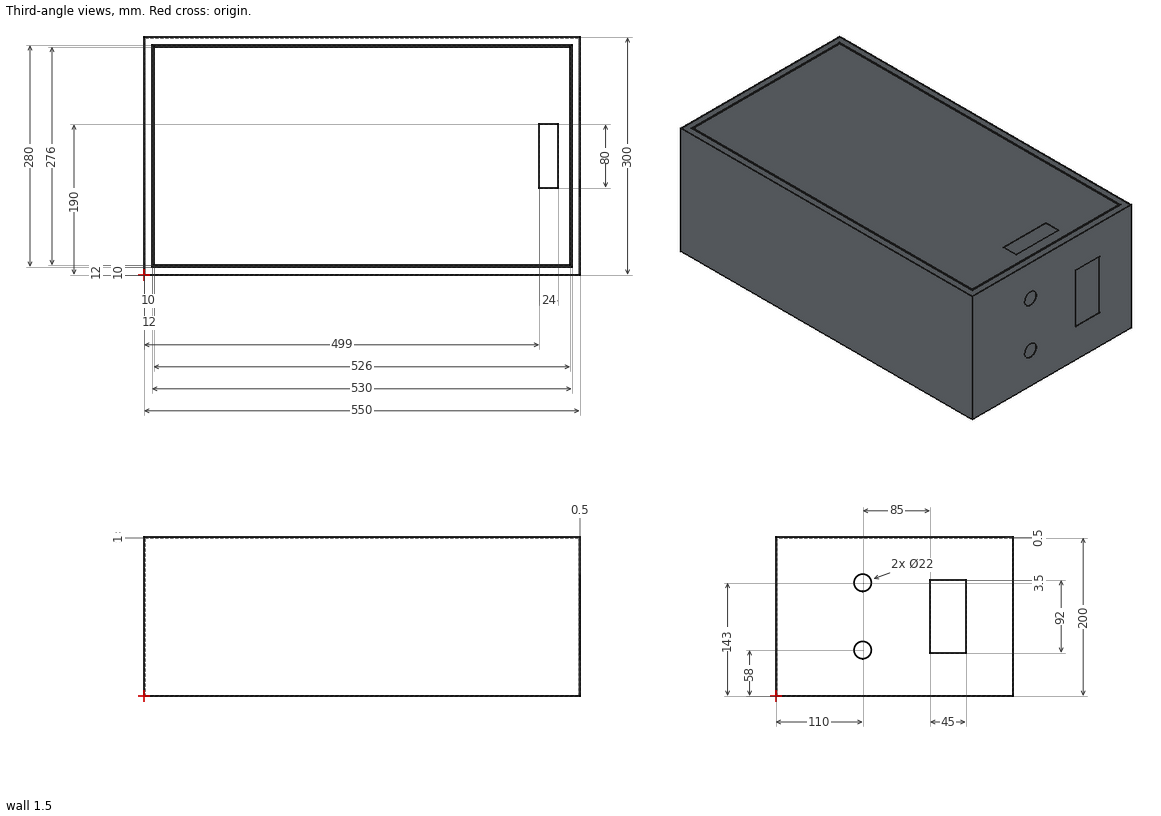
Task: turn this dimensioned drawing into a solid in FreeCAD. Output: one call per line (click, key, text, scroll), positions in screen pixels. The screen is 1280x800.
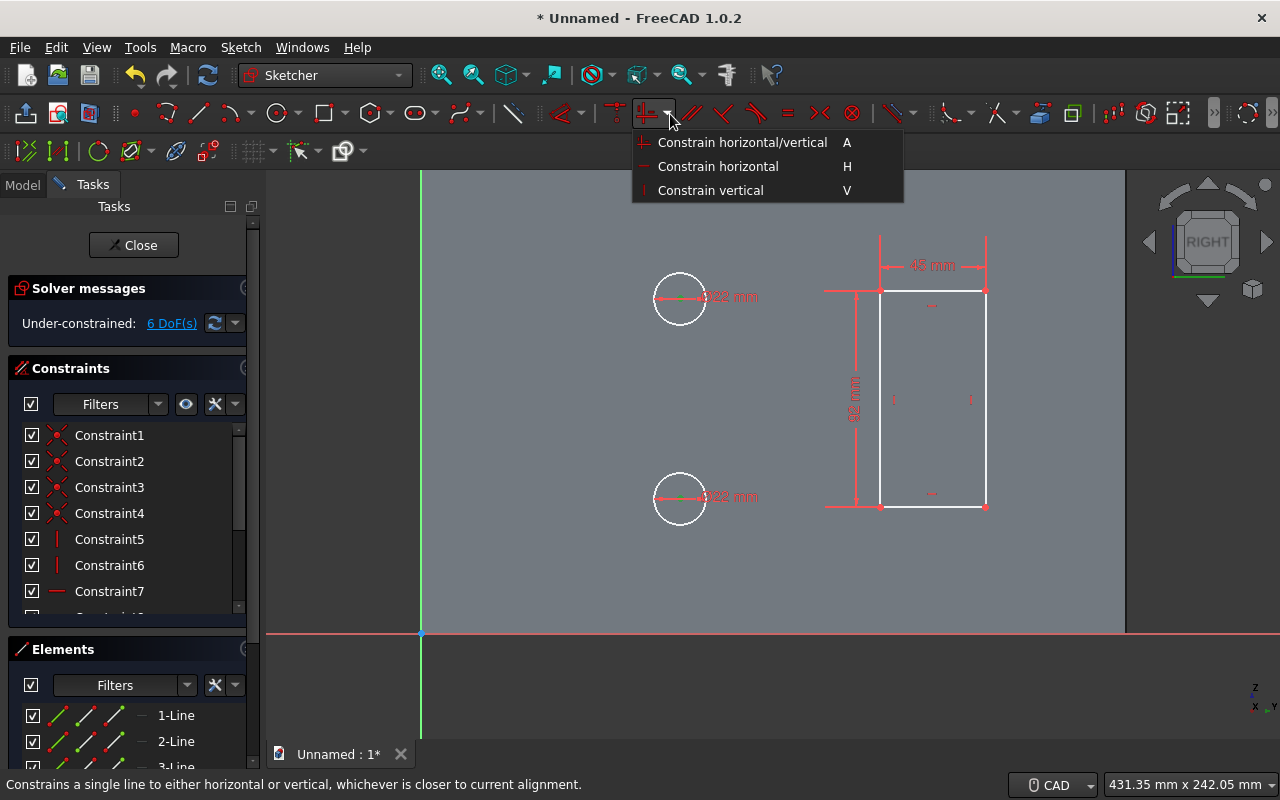
click(768, 190)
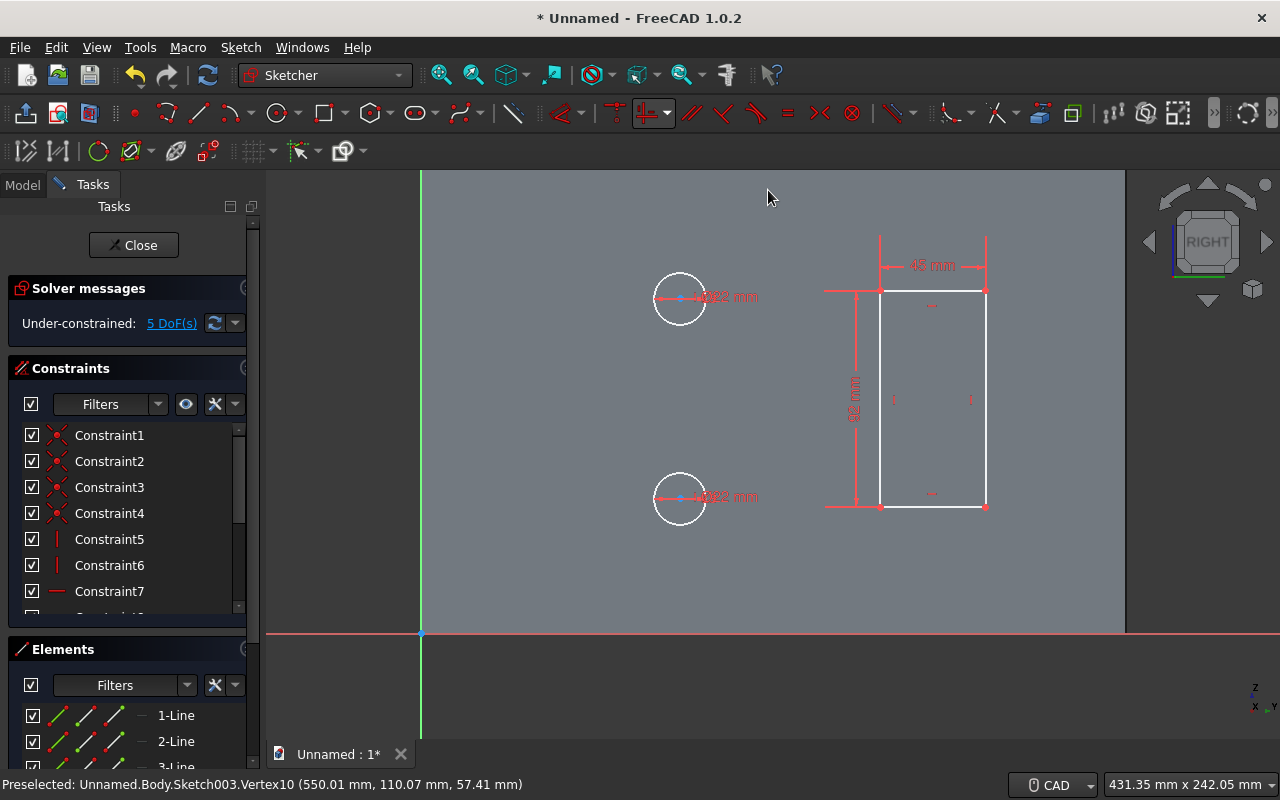
click(560, 114)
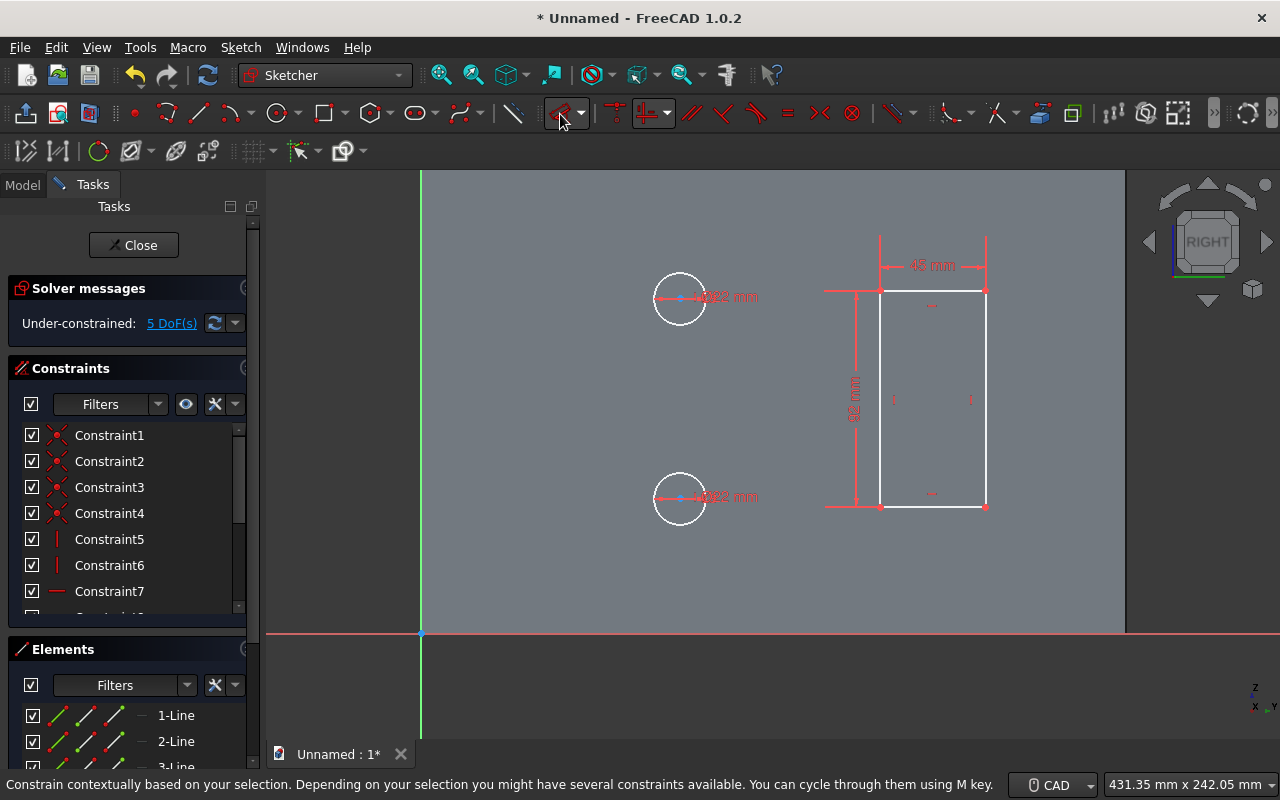
click(680, 499)
click(387, 566)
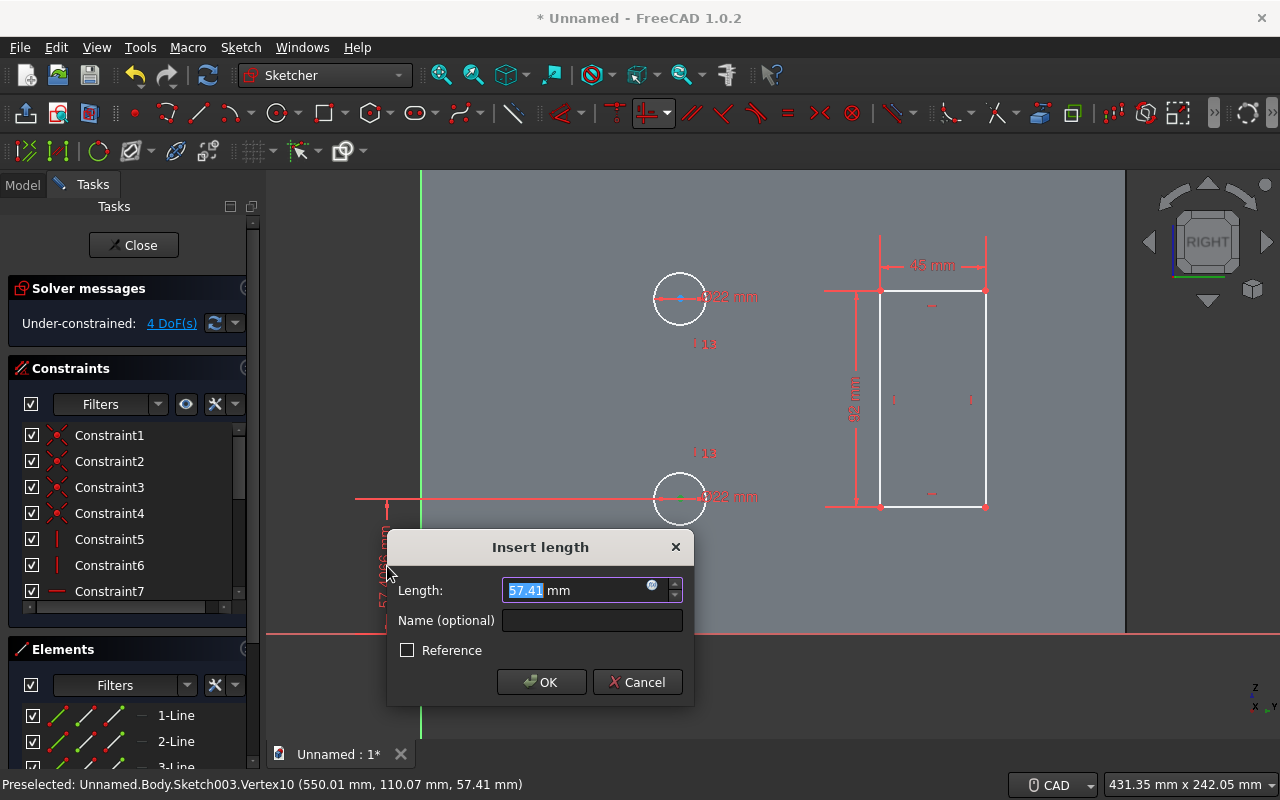
text(58)
key(Return)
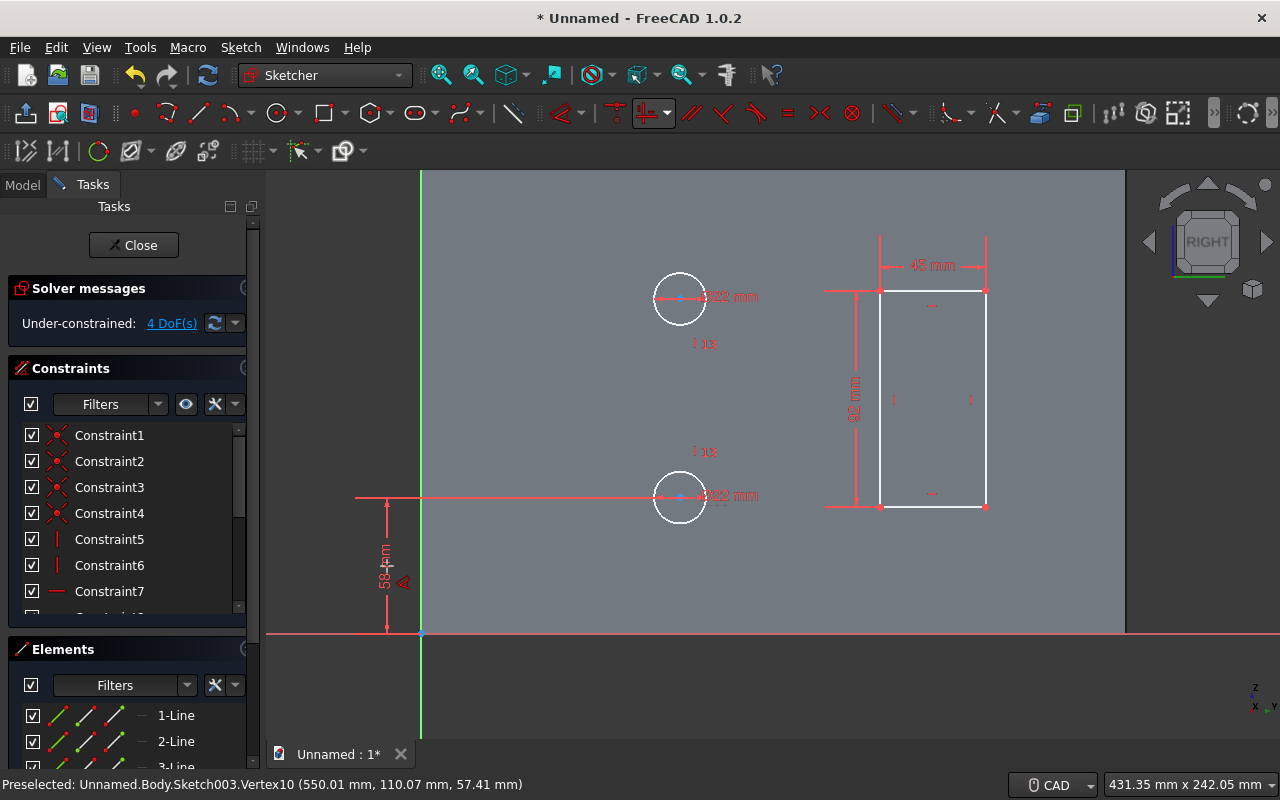
click(680, 299)
click(551, 668)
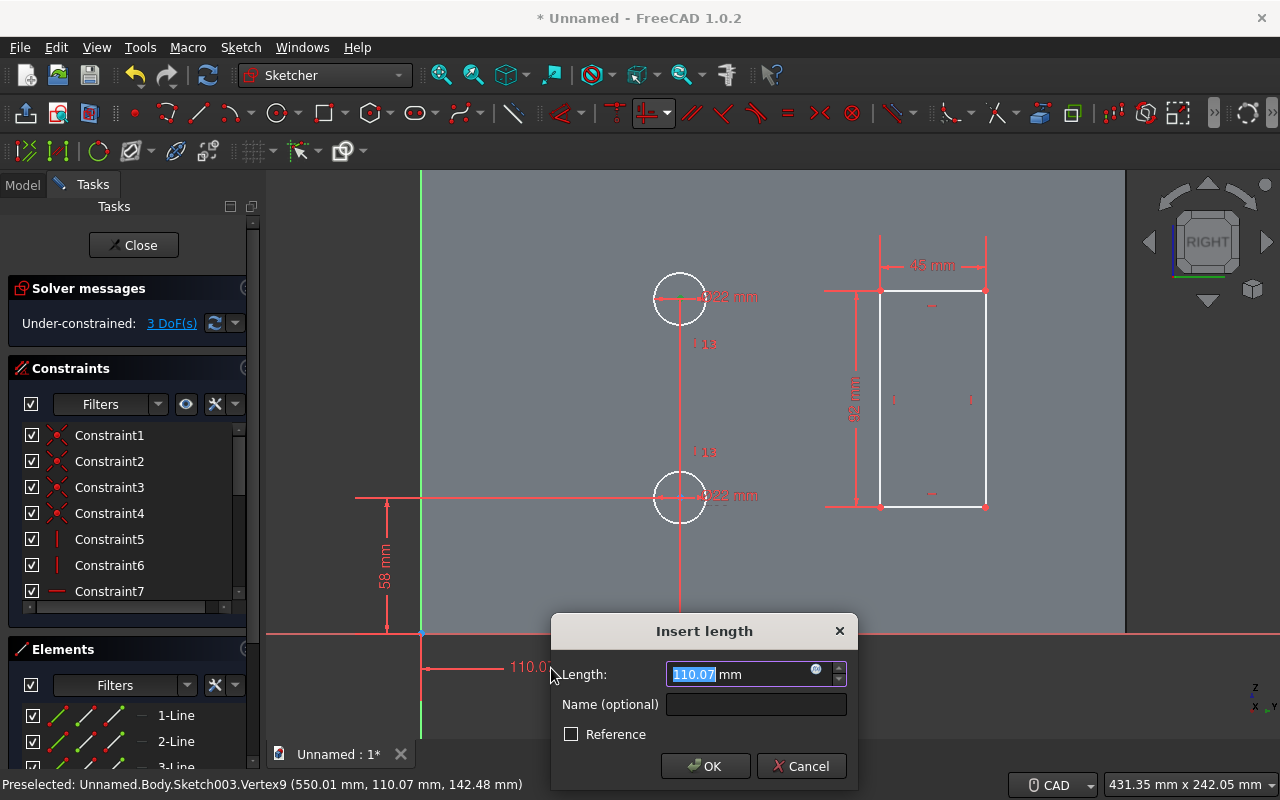
text(110)
key(Return)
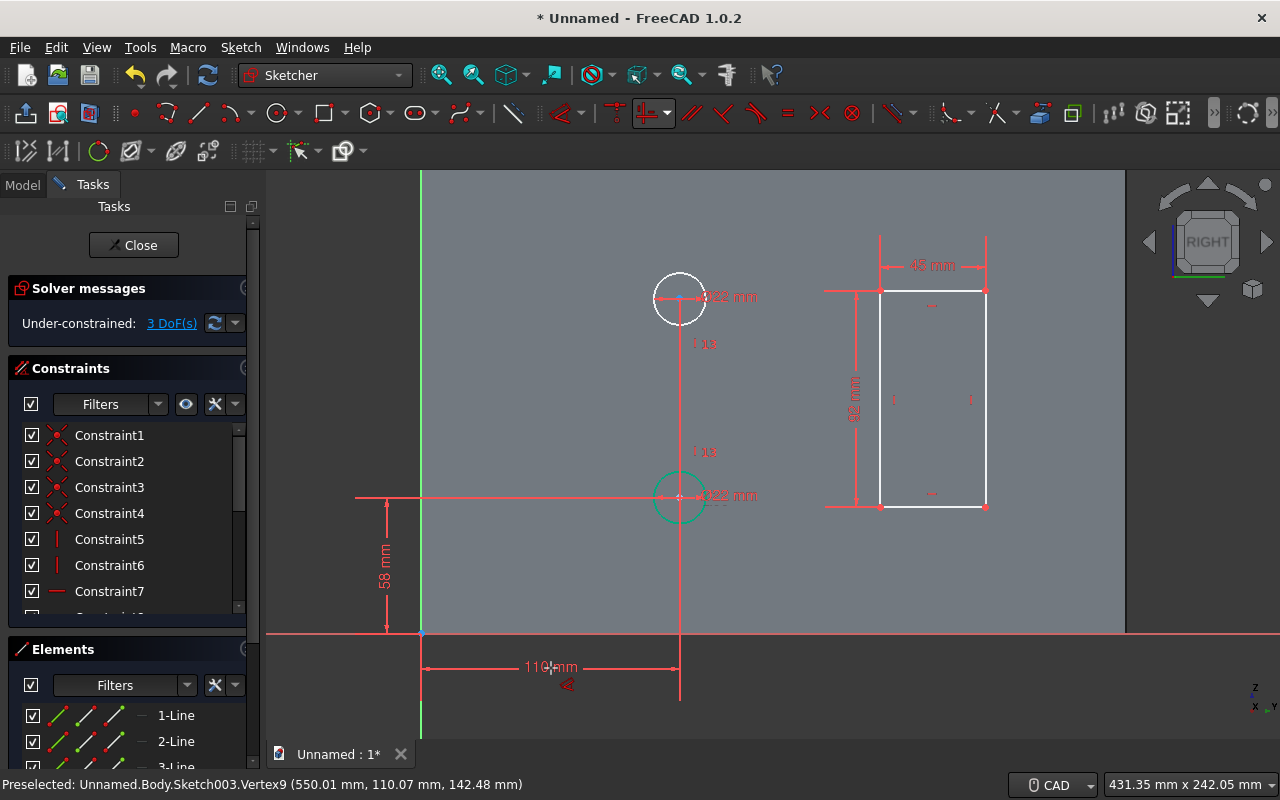
click(680, 299)
click(387, 466)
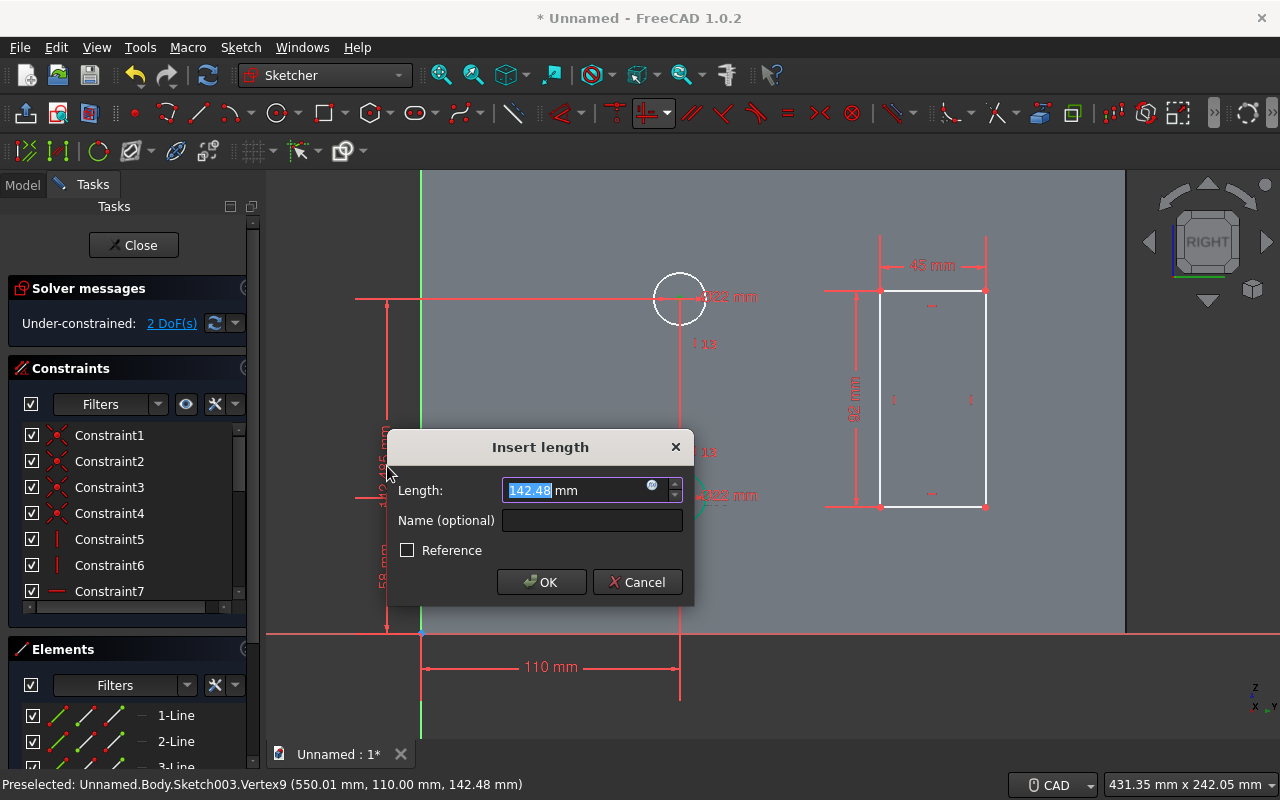
text(143)
key(Return)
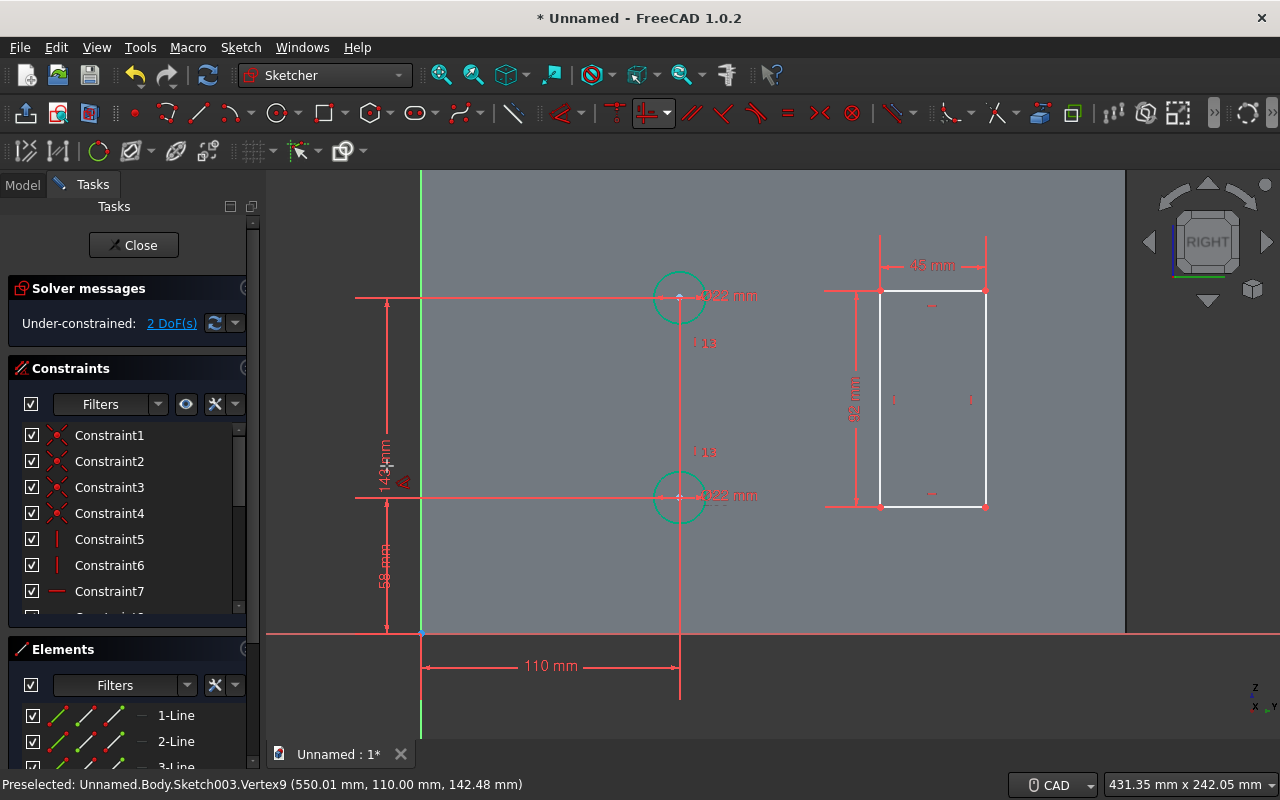
click(880, 291)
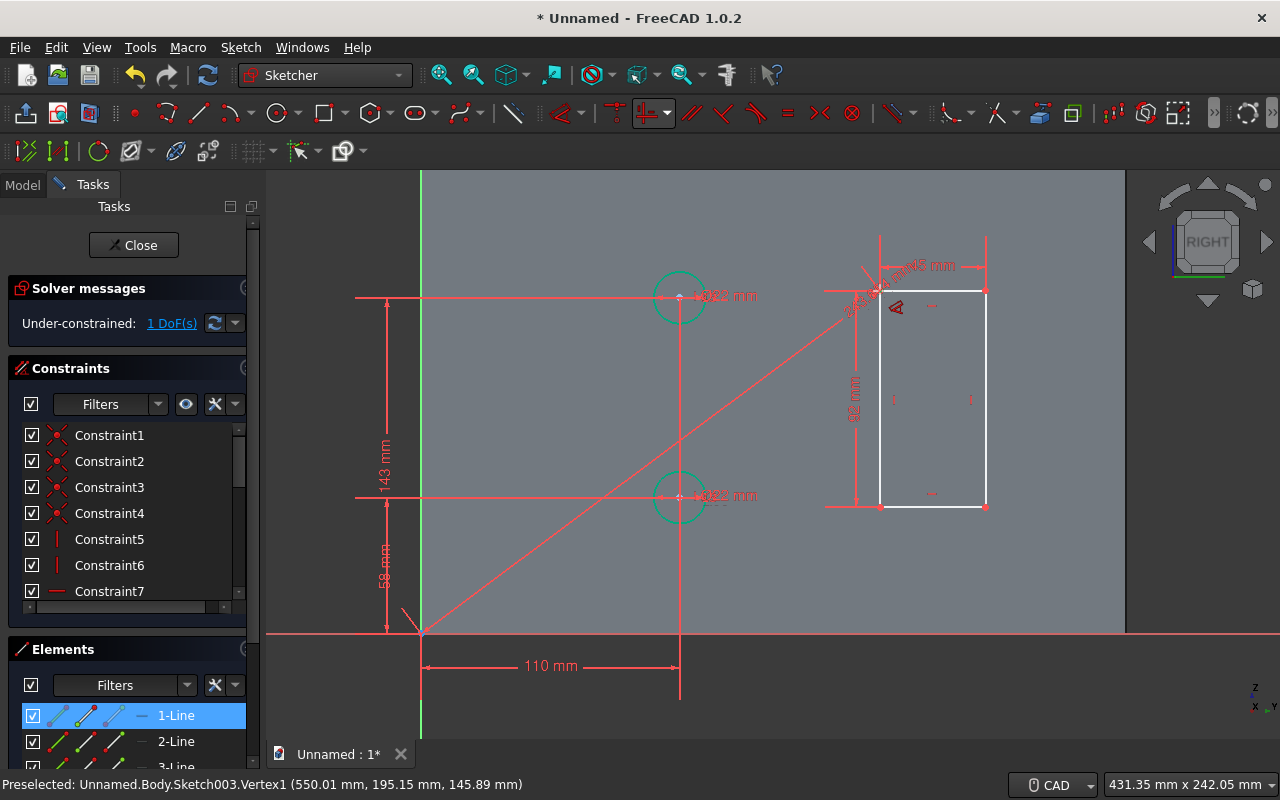
click(680, 298)
click(780, 257)